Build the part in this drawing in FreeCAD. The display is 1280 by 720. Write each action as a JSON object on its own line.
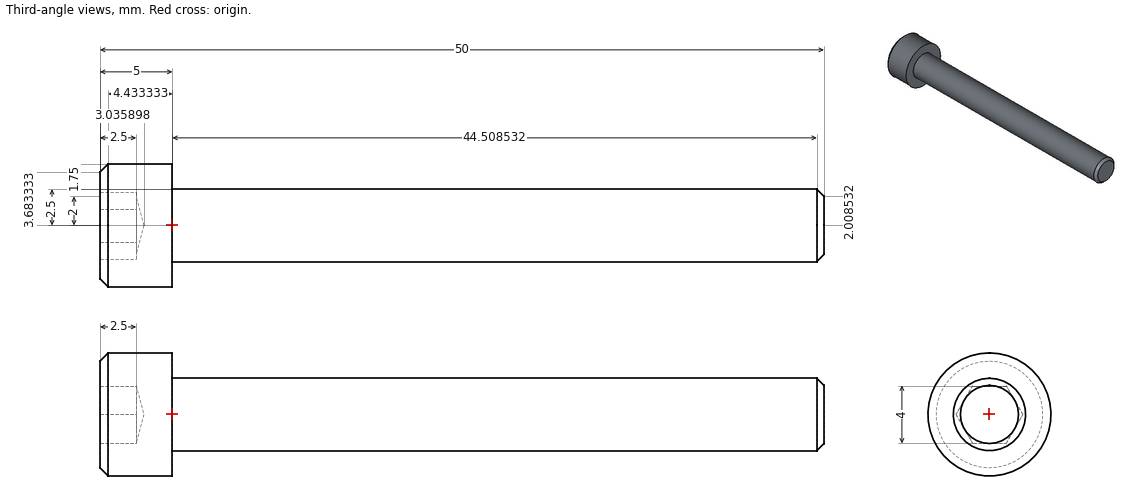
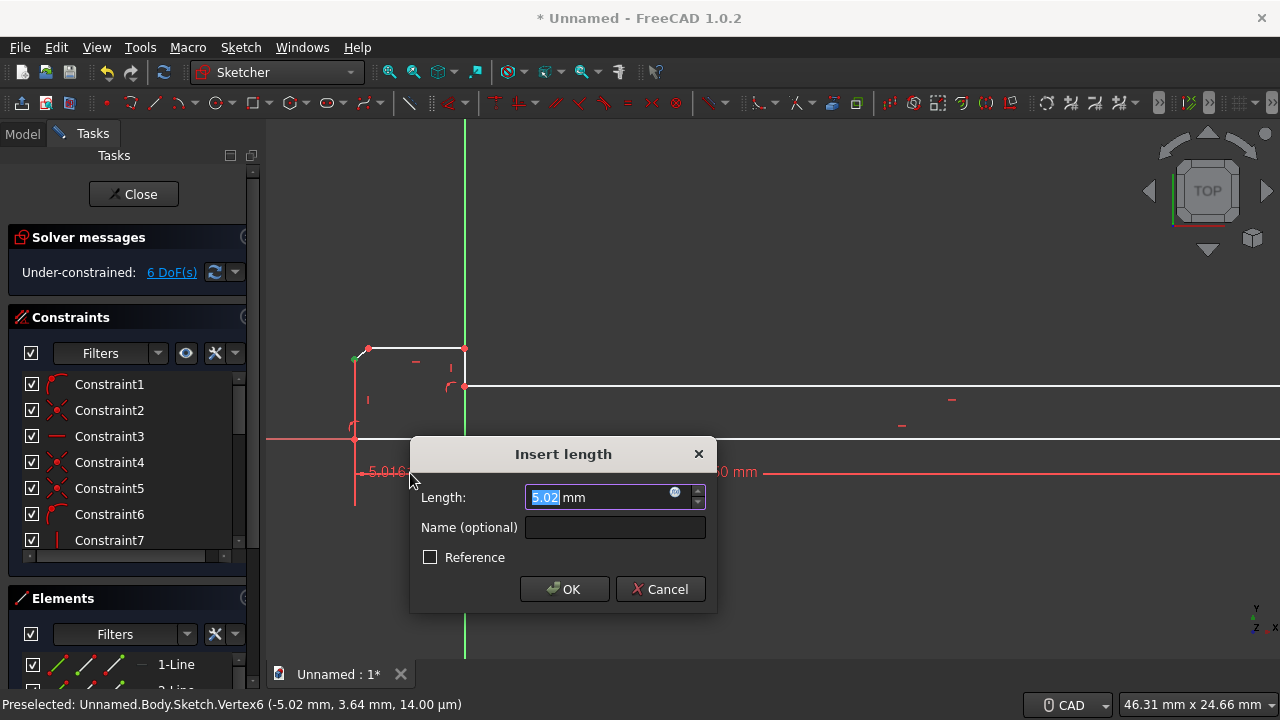
{"action": "type", "text": "5"}
{"action": "key", "text": "Return"}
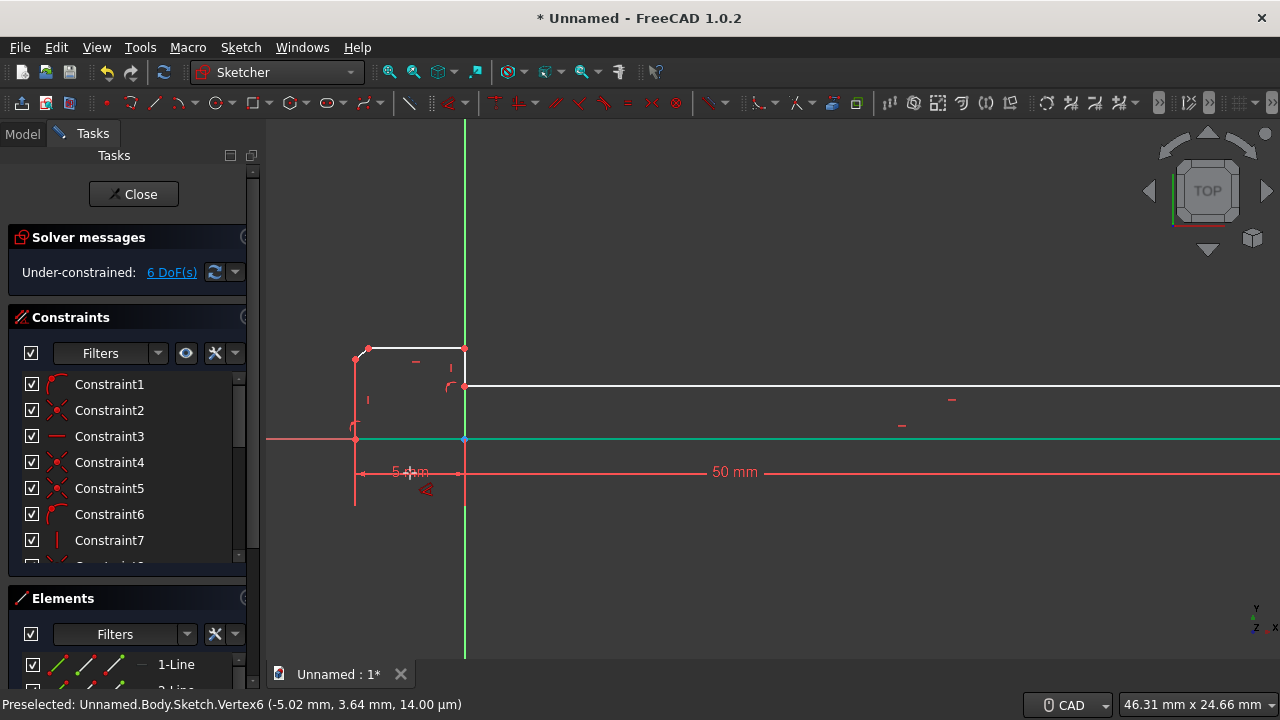
{"action": "left_click", "coordinate": [465, 375]}
{"action": "left_click", "coordinate": [431, 367]}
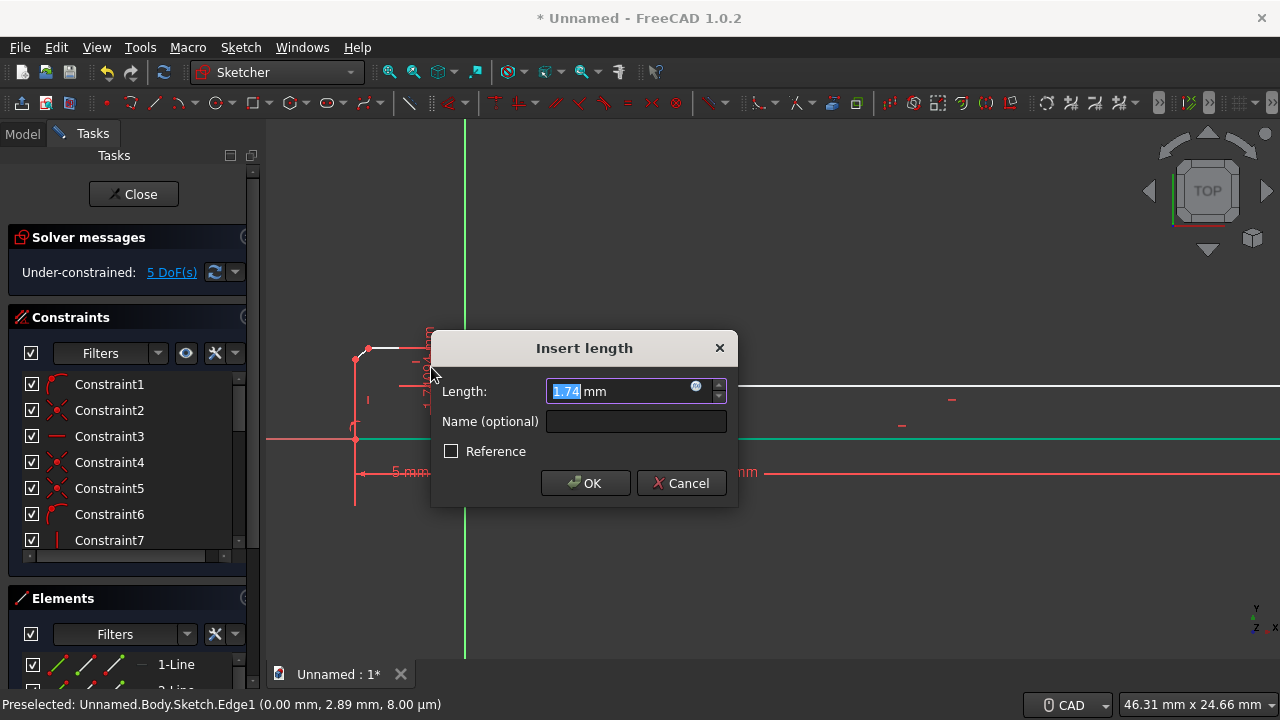
{"action": "type", "text": "1.75"}
{"action": "key", "text": "Return"}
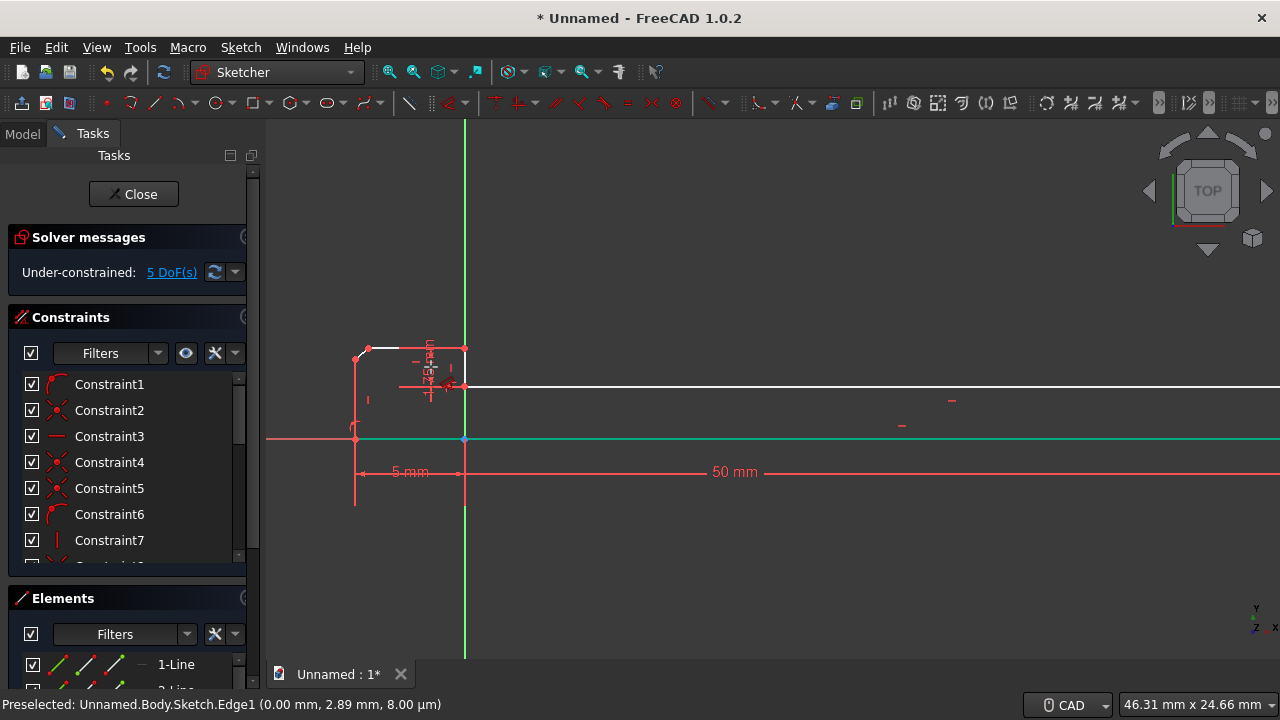
{"action": "left_click", "coordinate": [465, 387]}
{"action": "left_click", "coordinate": [431, 413]}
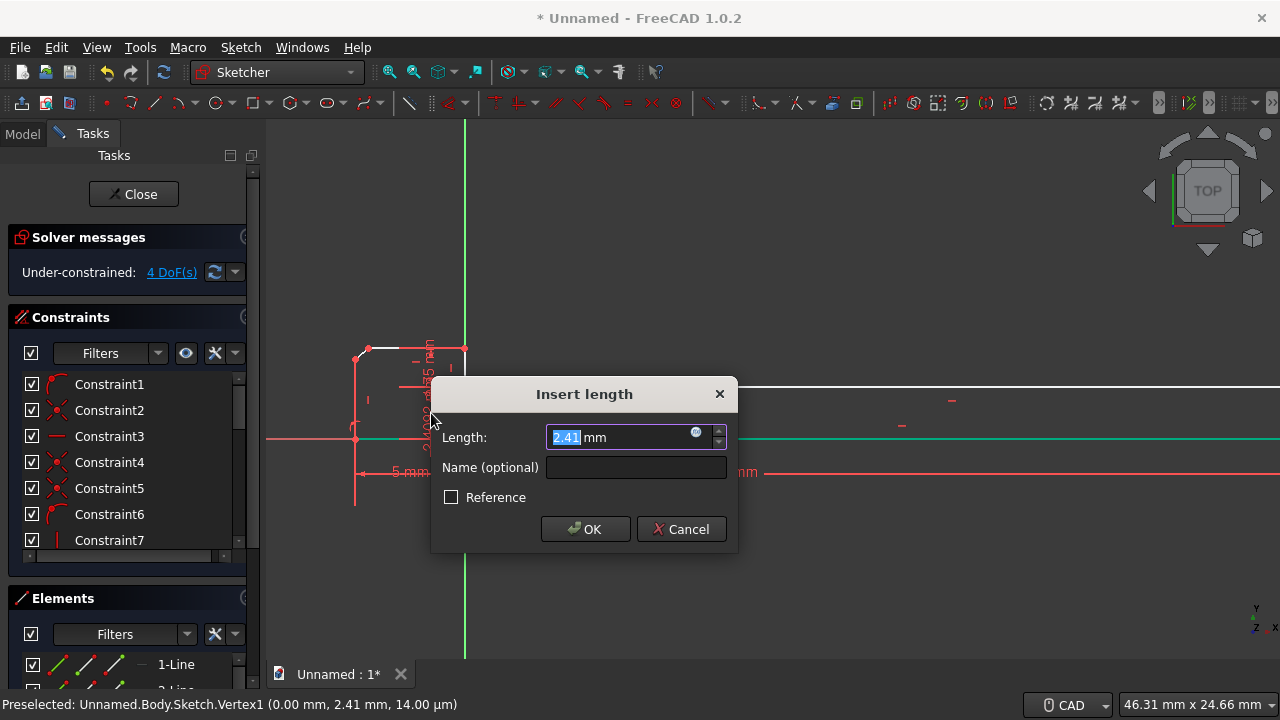
{"action": "type", "text": "2.5"}
{"action": "key", "text": "Return"}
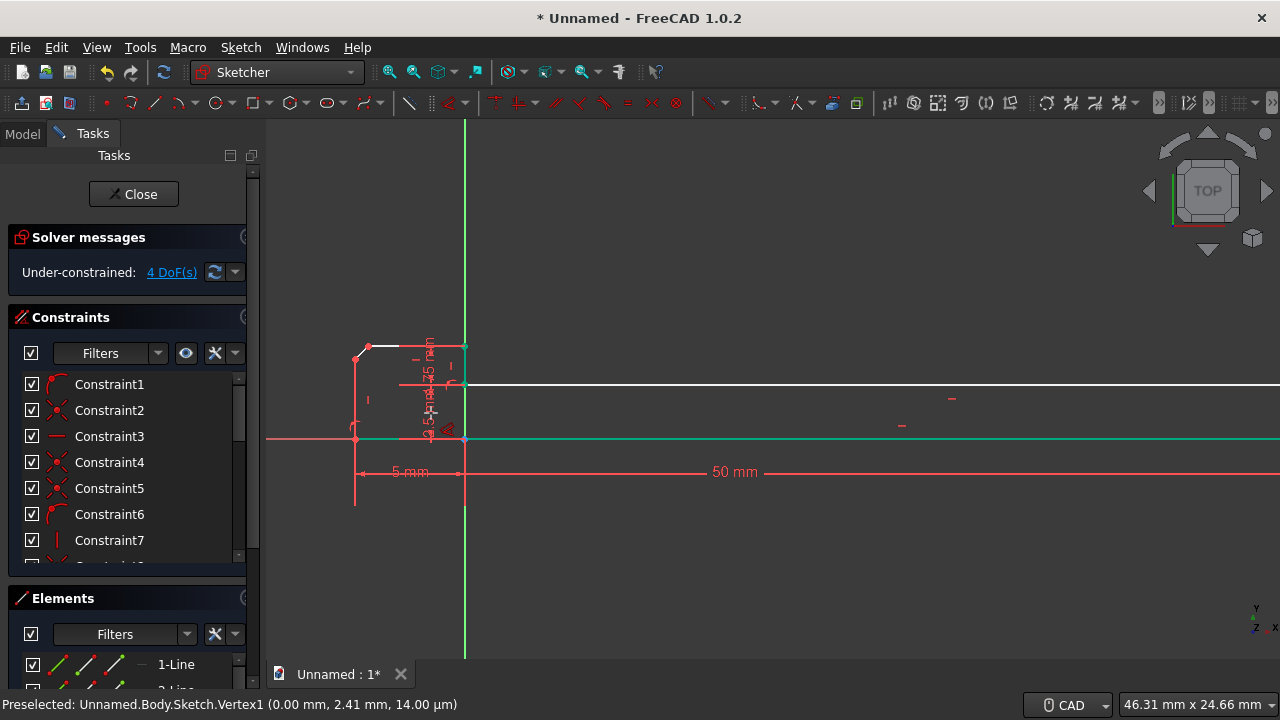
{"action": "left_click", "coordinate": [436, 346]}
{"action": "left_click", "coordinate": [417, 312]}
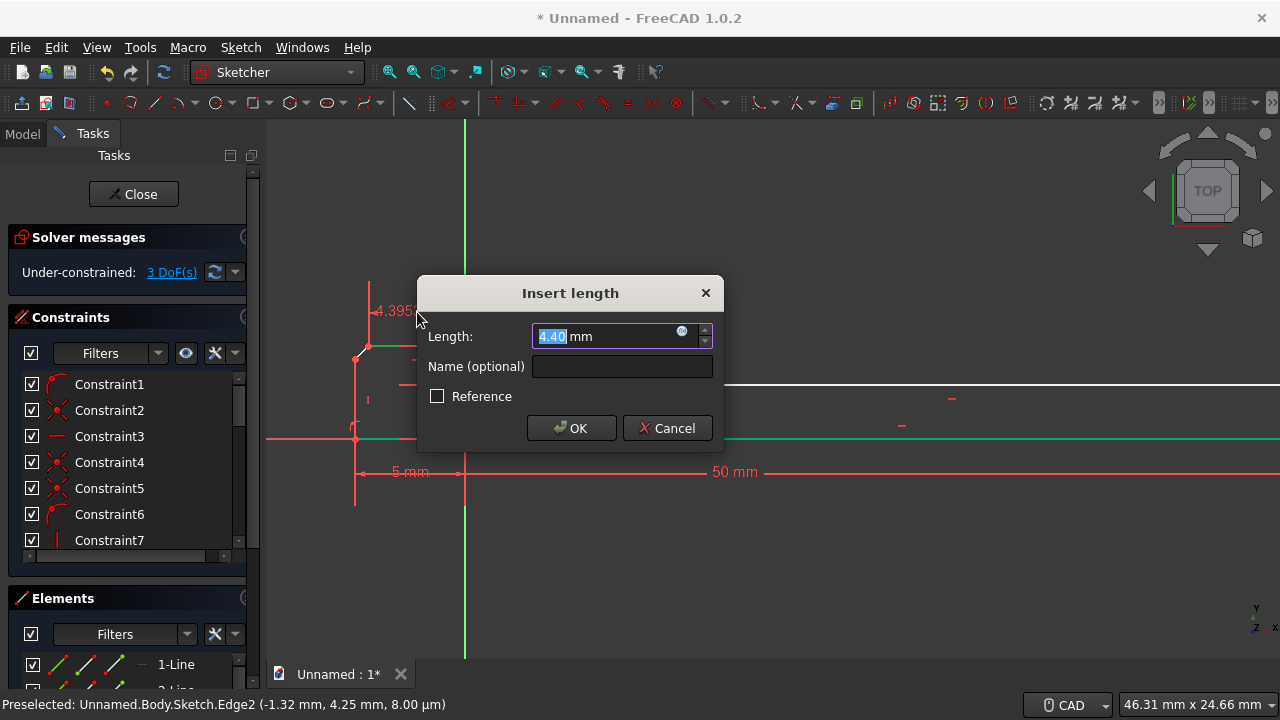
{"action": "type", "text": "4.433333"}
{"action": "key", "text": "Return"}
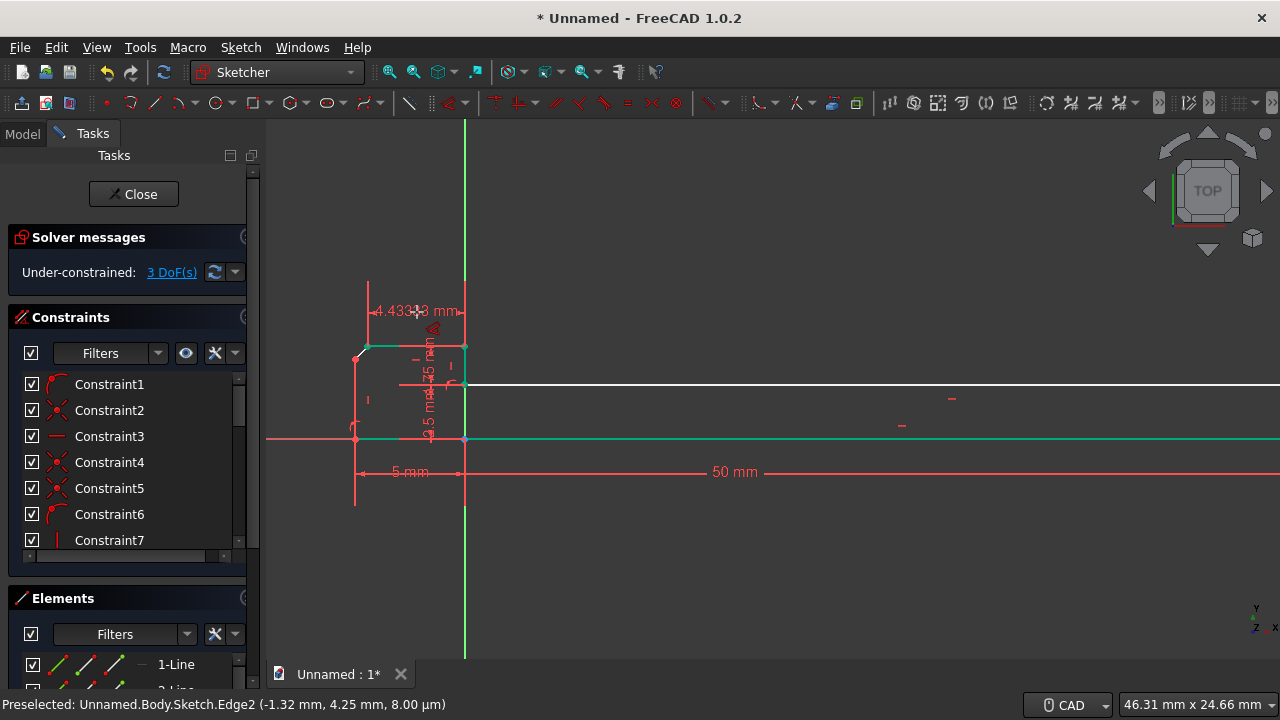
{"action": "left_click", "coordinate": [355, 384]}
{"action": "left_click", "coordinate": [321, 399]}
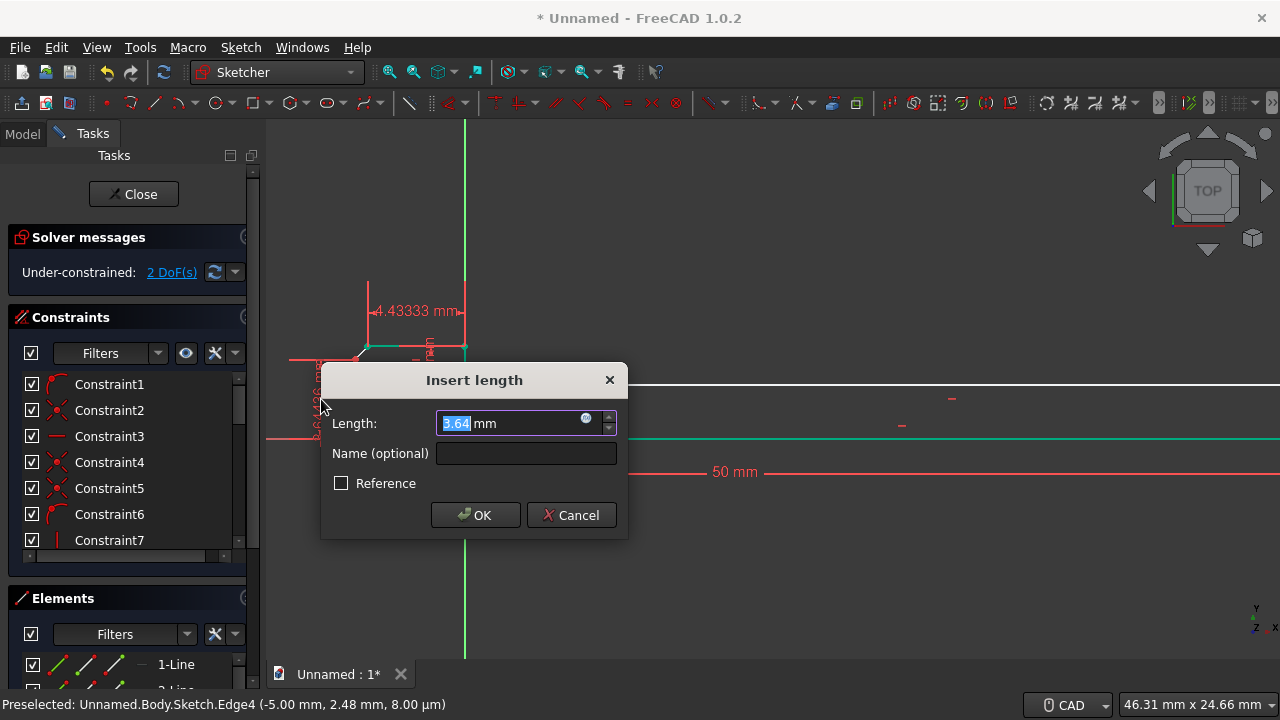
{"action": "type", "text": "3.683333"}
{"action": "key", "text": "Return"}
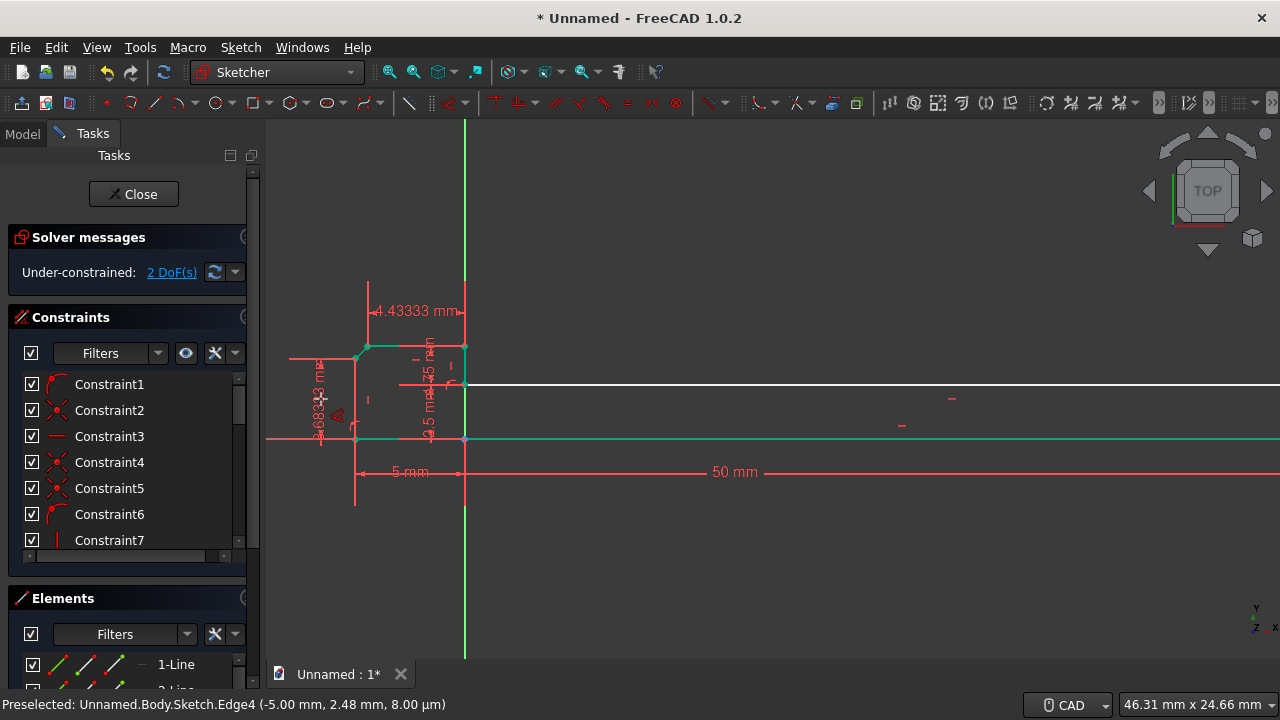
{"action": "scroll", "coordinate": [463, 384], "scroll_direction": "down", "scroll_amount": 3}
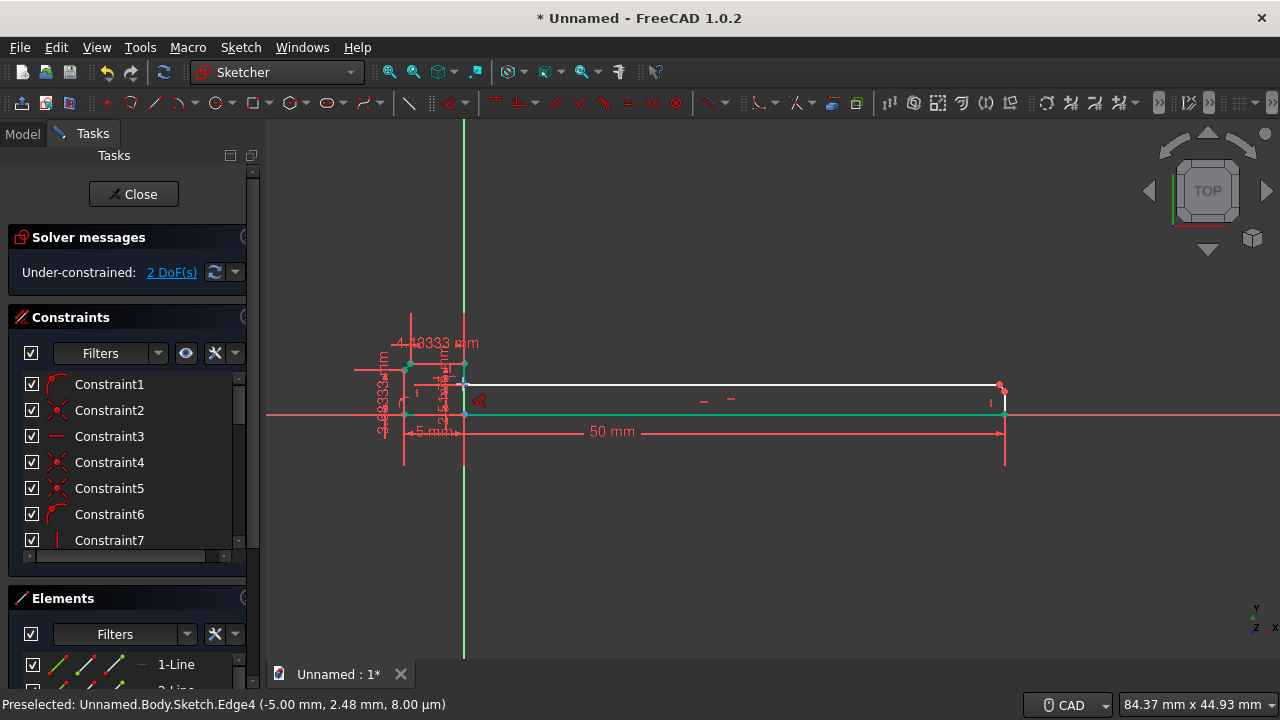
{"action": "scroll", "coordinate": [1005, 408], "scroll_direction": "up", "scroll_amount": 4}